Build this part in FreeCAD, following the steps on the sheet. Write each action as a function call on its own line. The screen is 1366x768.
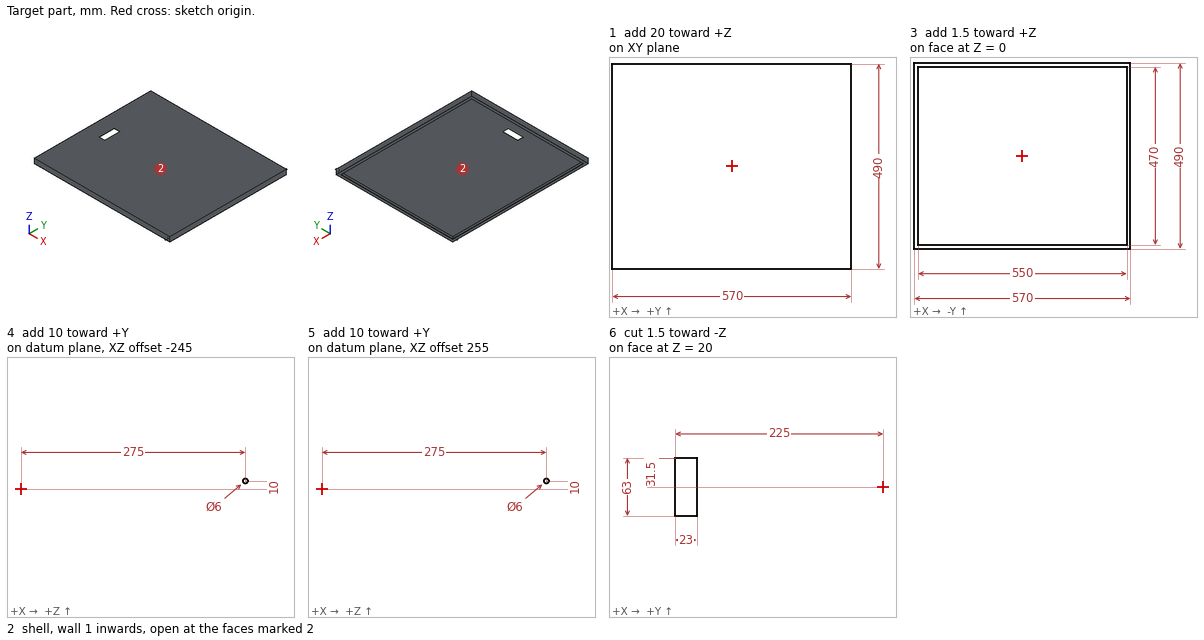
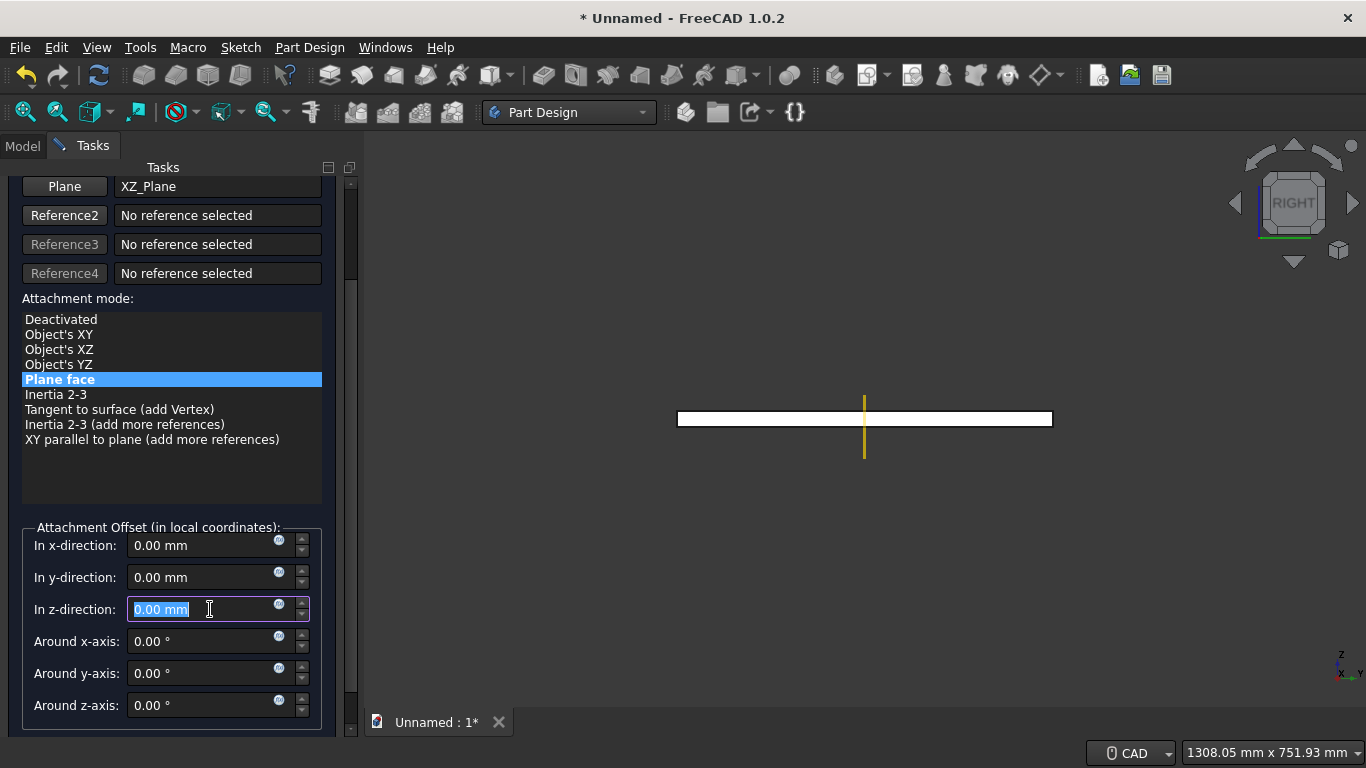
text(-245)
key(Tab)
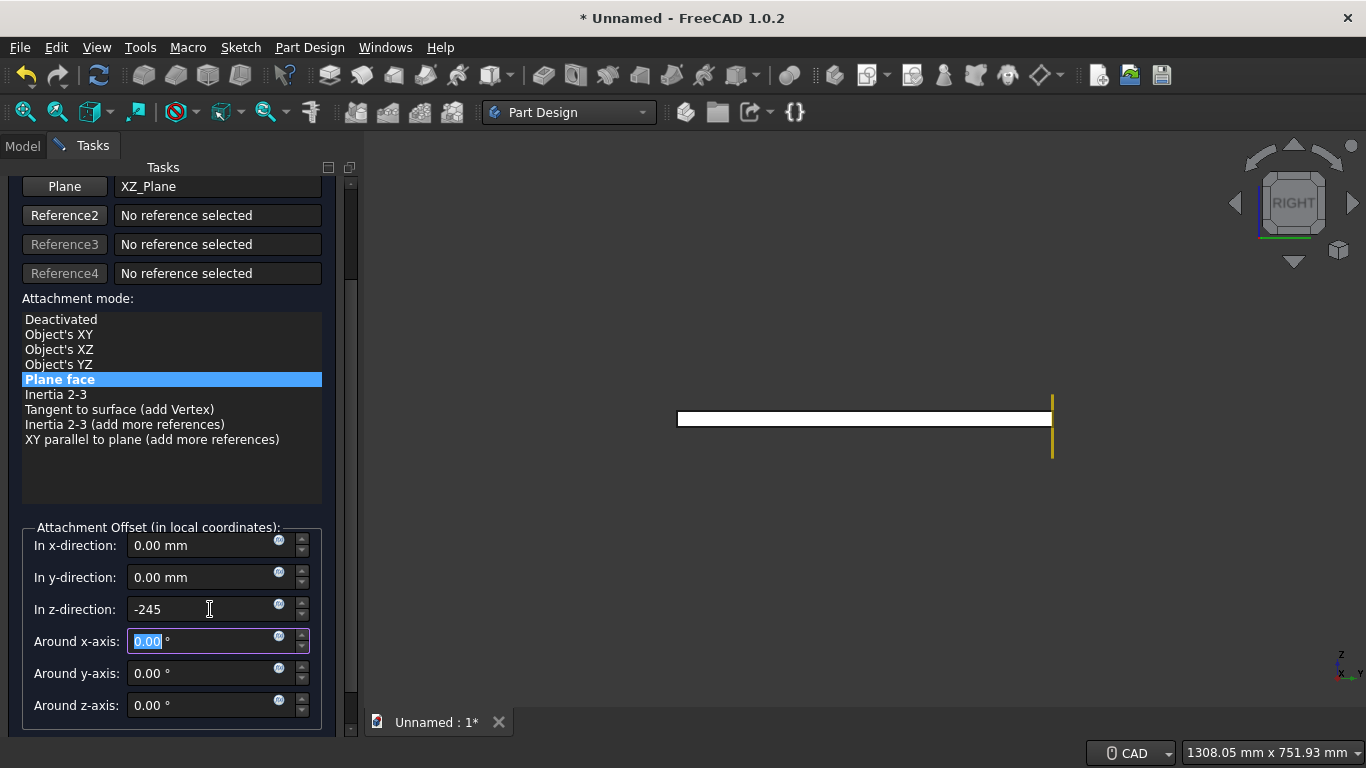
scroll(351, 456, up, 3)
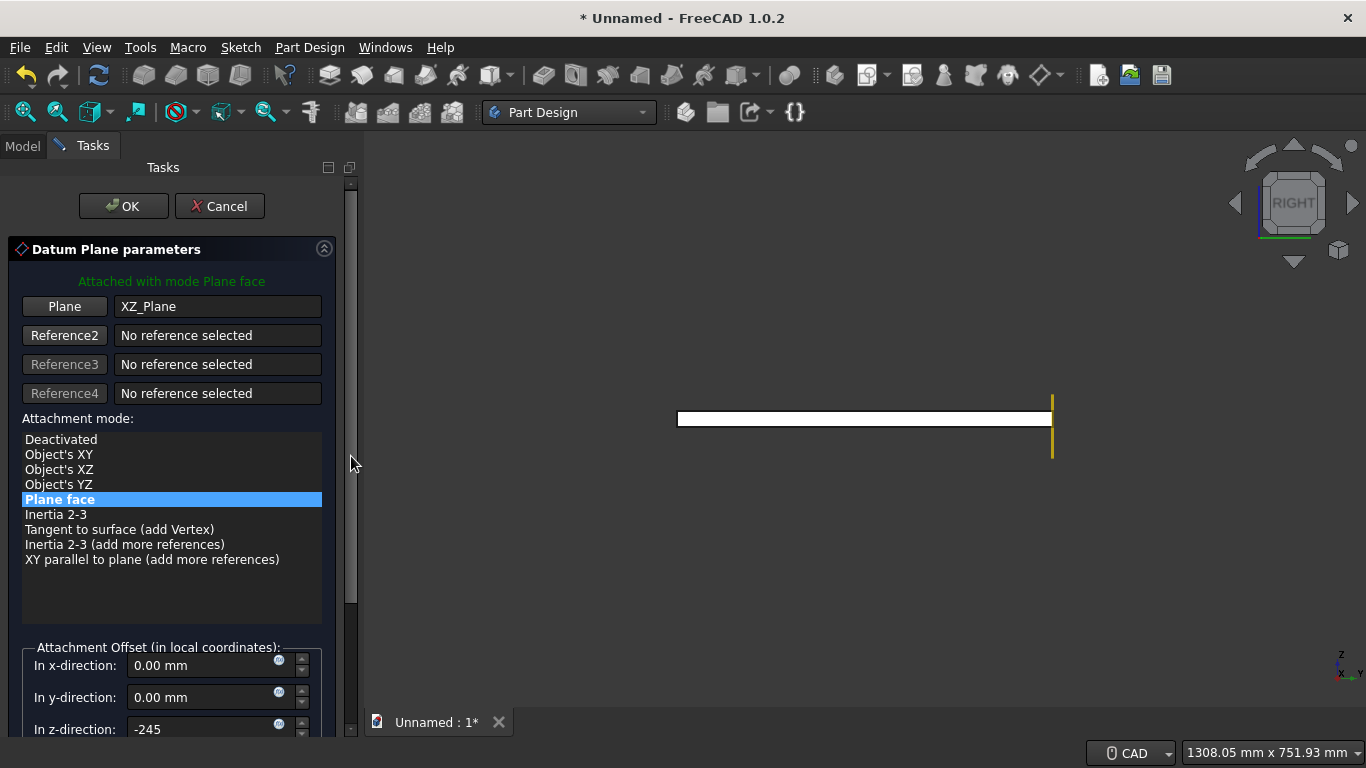
click(124, 206)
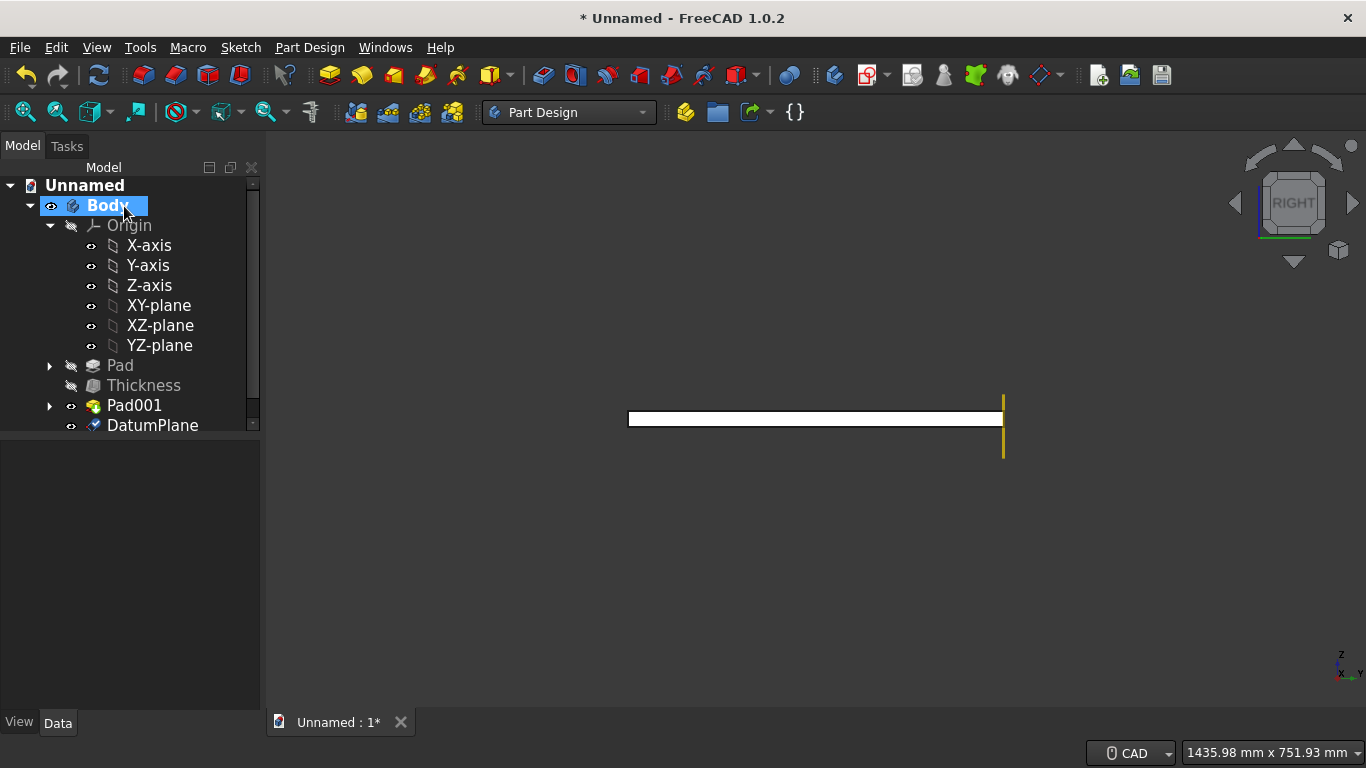
click(116, 426)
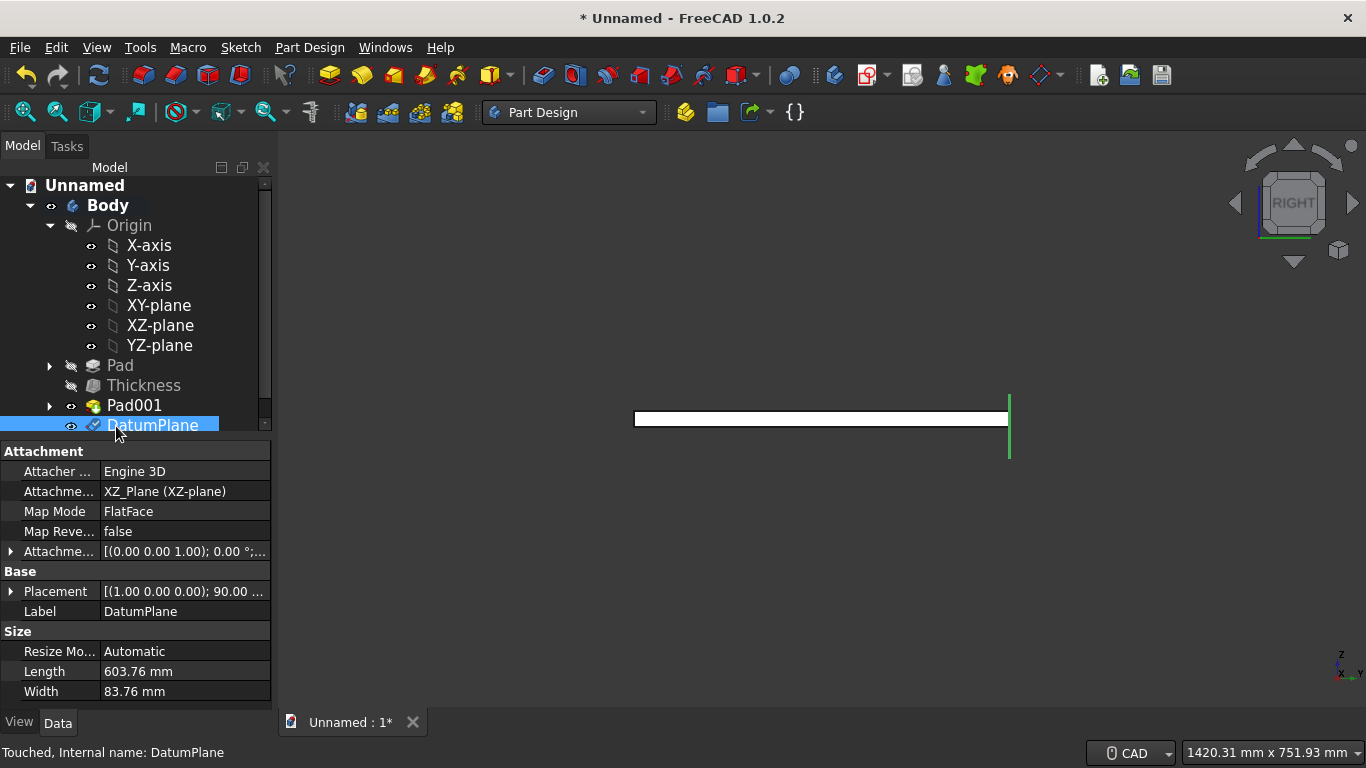
click(868, 76)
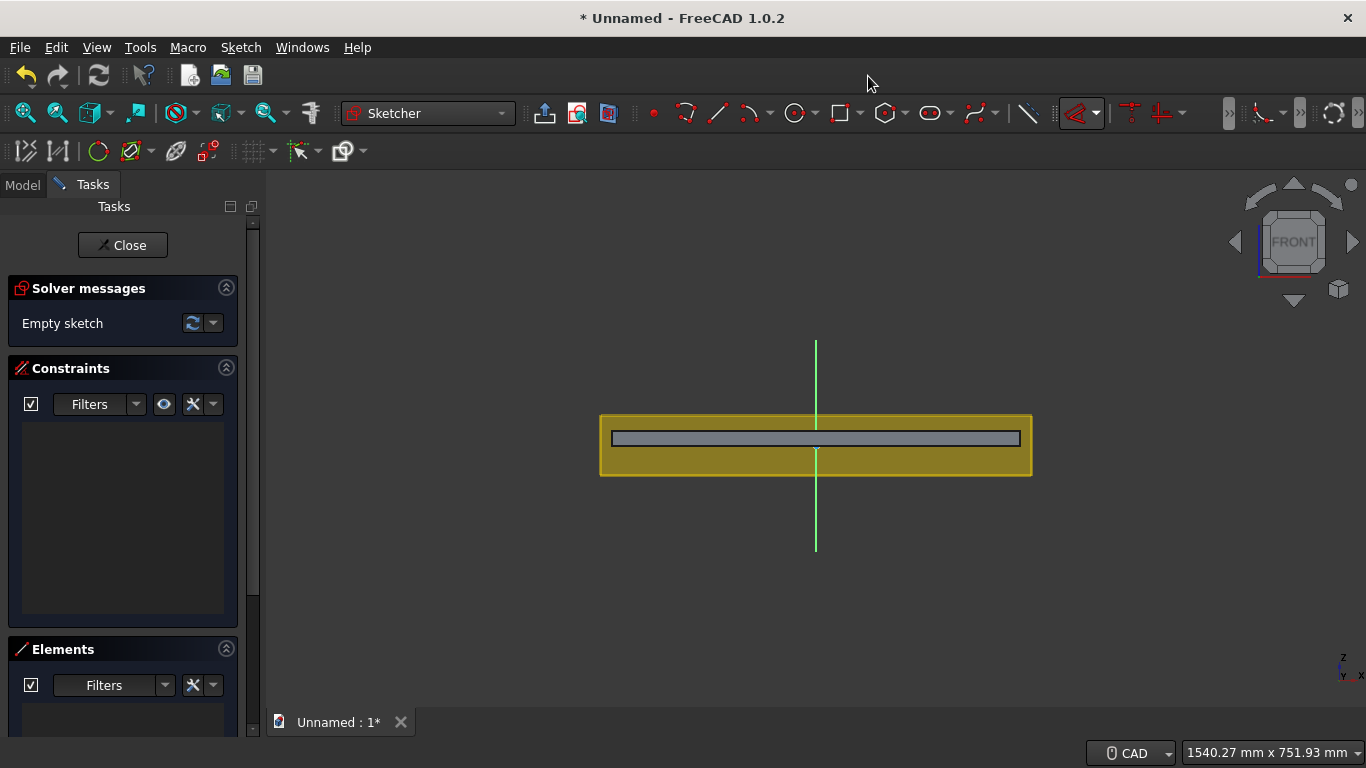
key(q)
key(s)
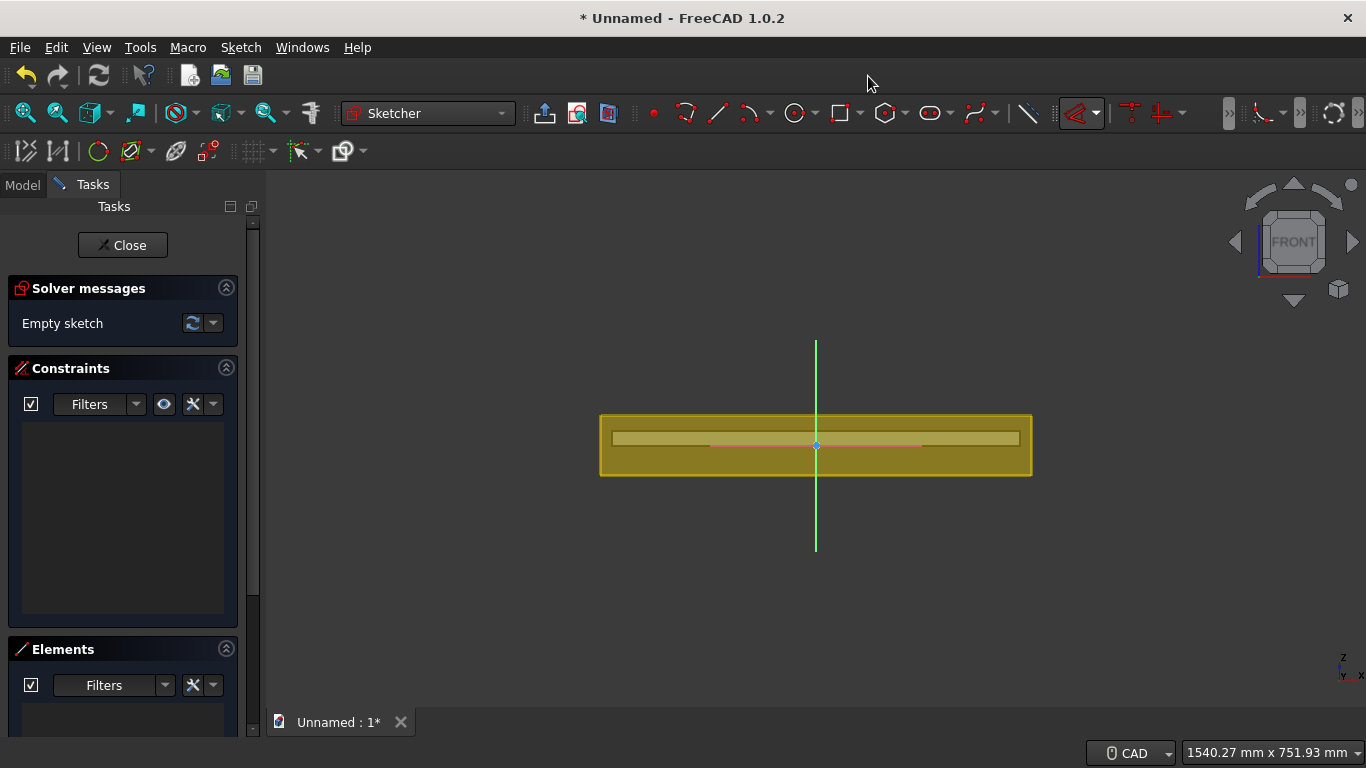
scroll(1026, 439, up, 15)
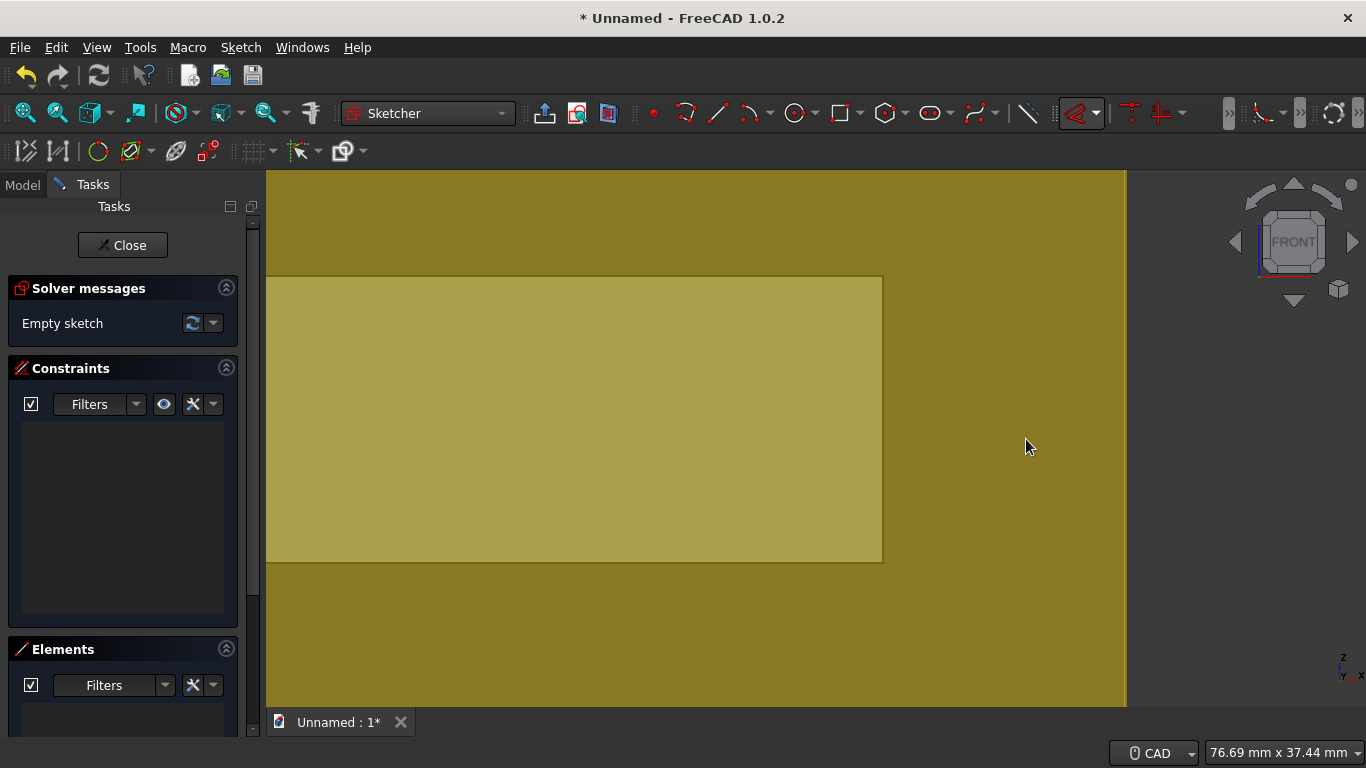
scroll(737, 413, up, 7)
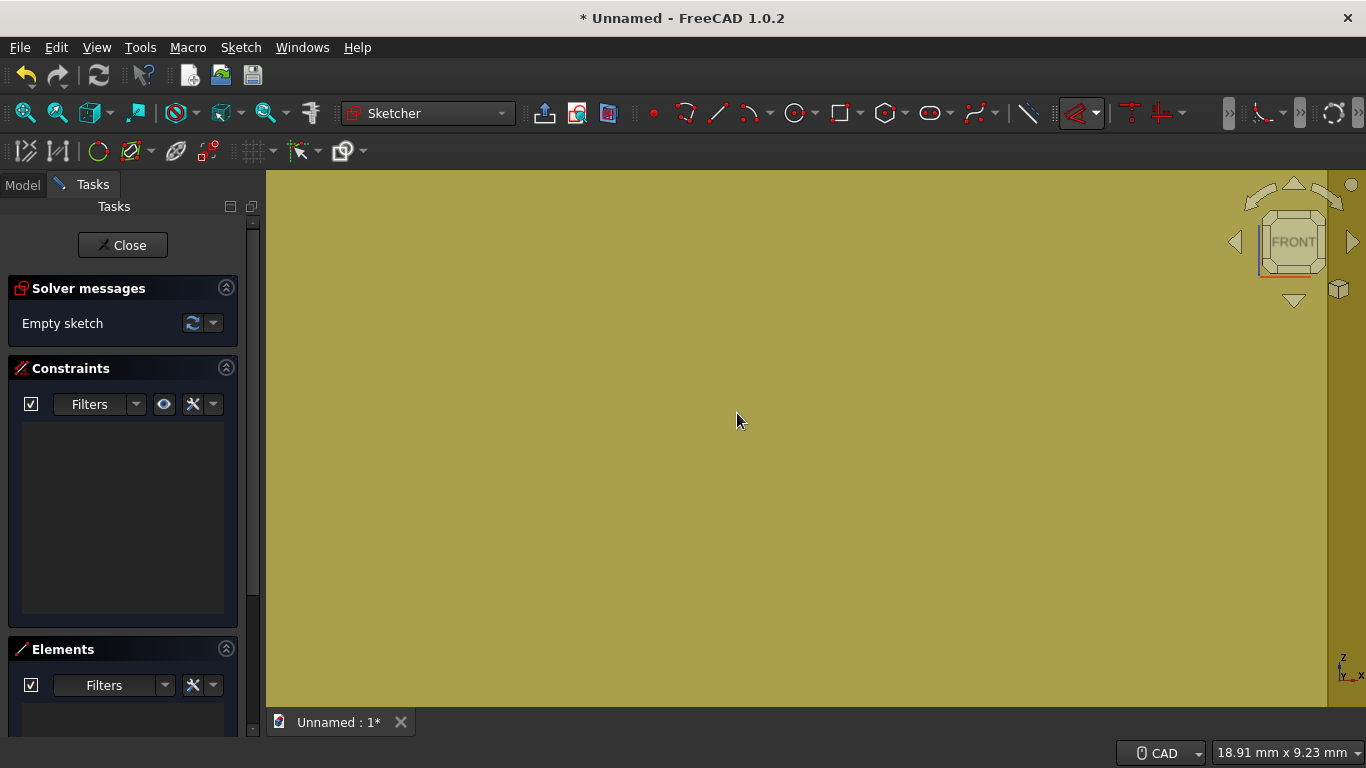
key(g)
key(c)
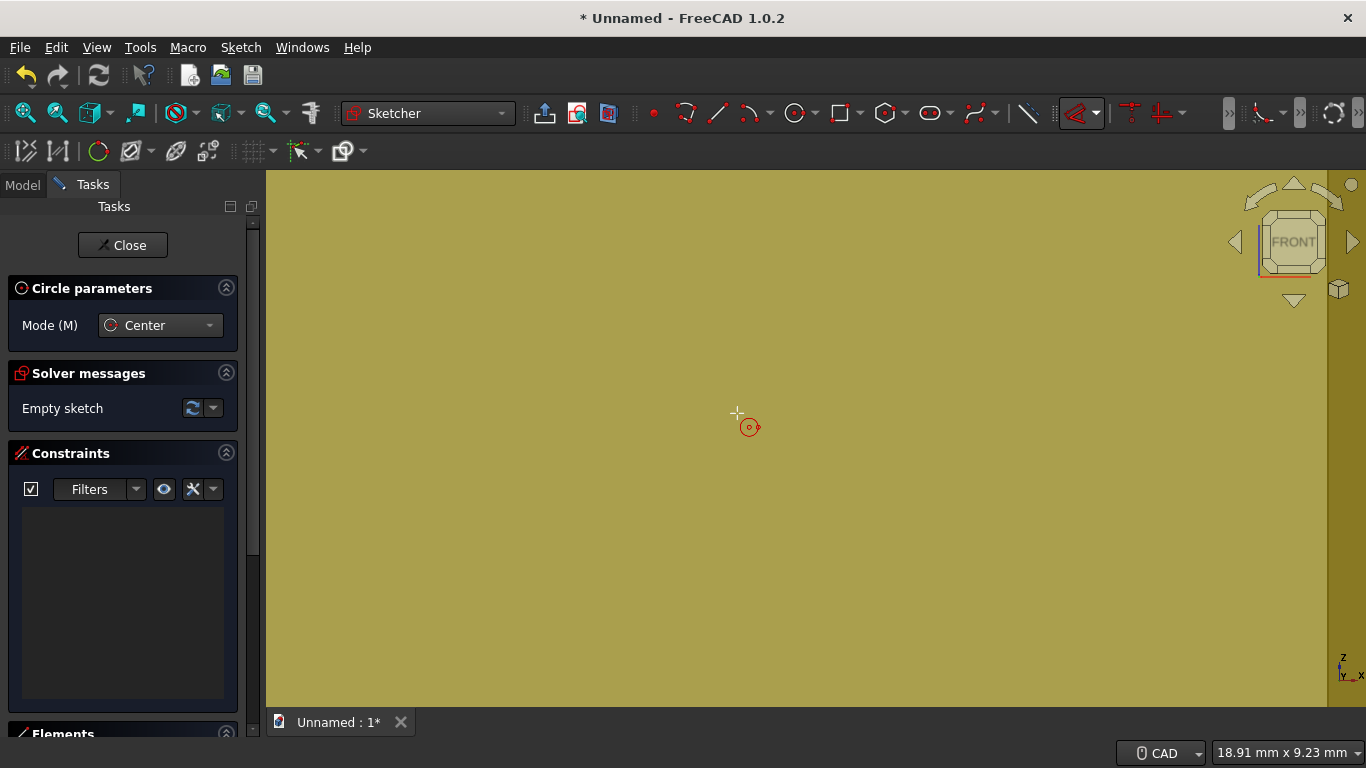
click(746, 437)
click(869, 314)
key(Escape)